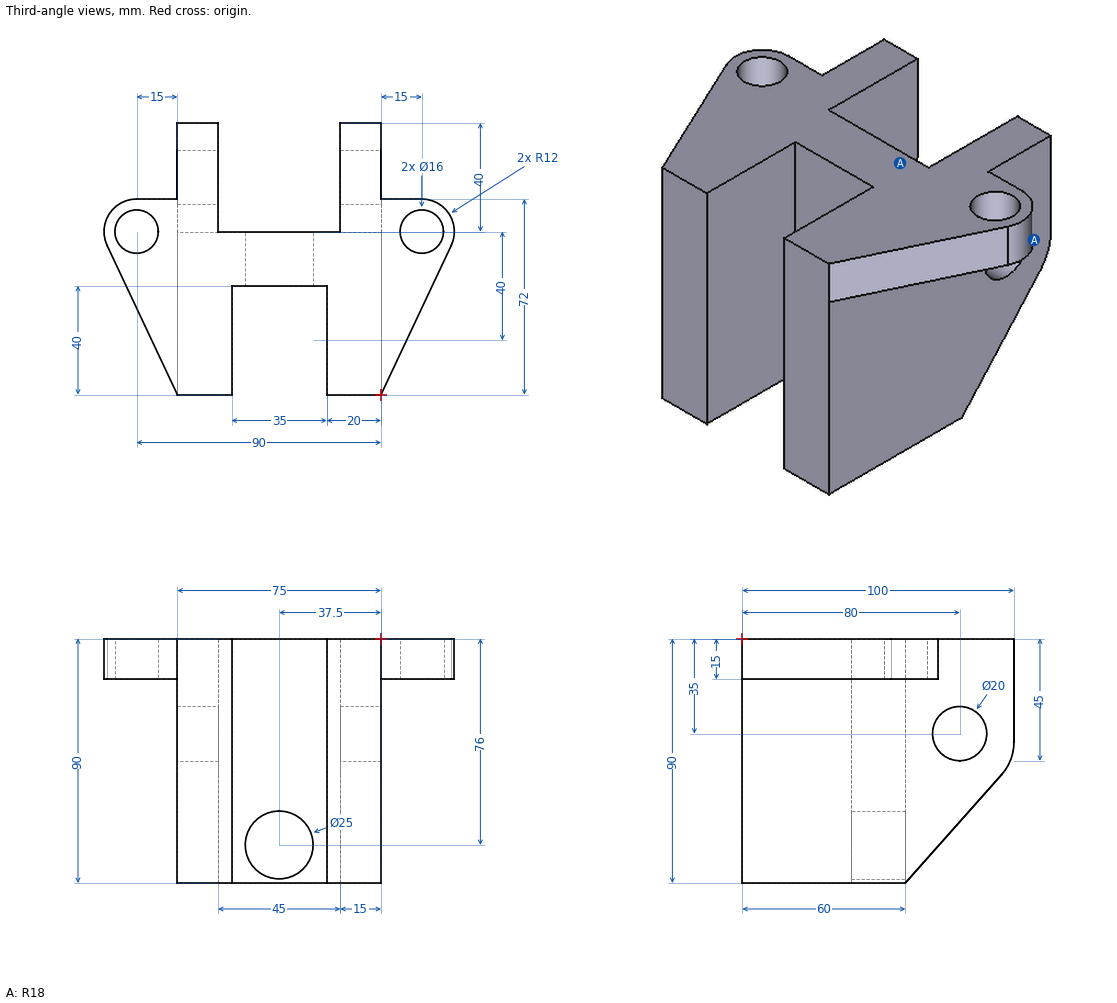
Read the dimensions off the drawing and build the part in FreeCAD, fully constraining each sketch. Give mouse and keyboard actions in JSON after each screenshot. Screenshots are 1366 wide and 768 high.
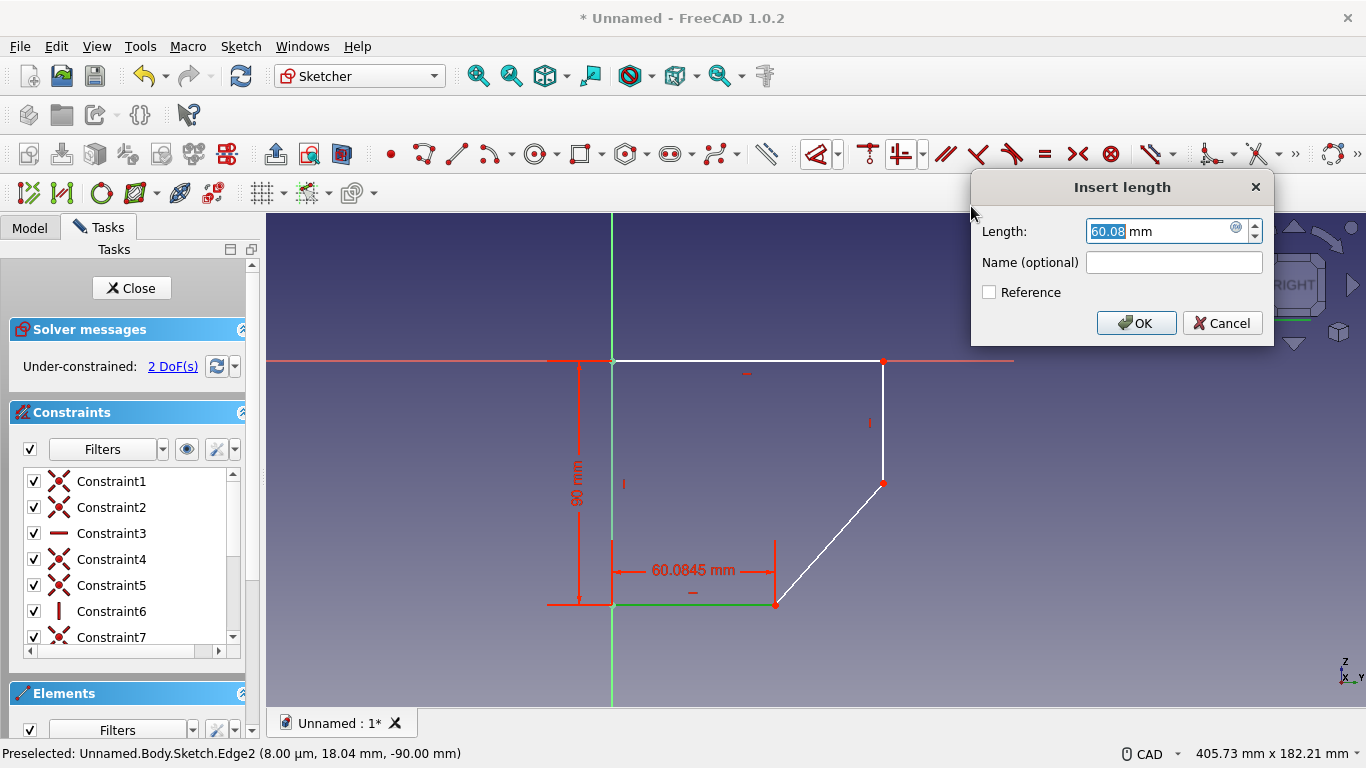
{"action": "type", "text": "60"}
{"action": "key", "text": "Return"}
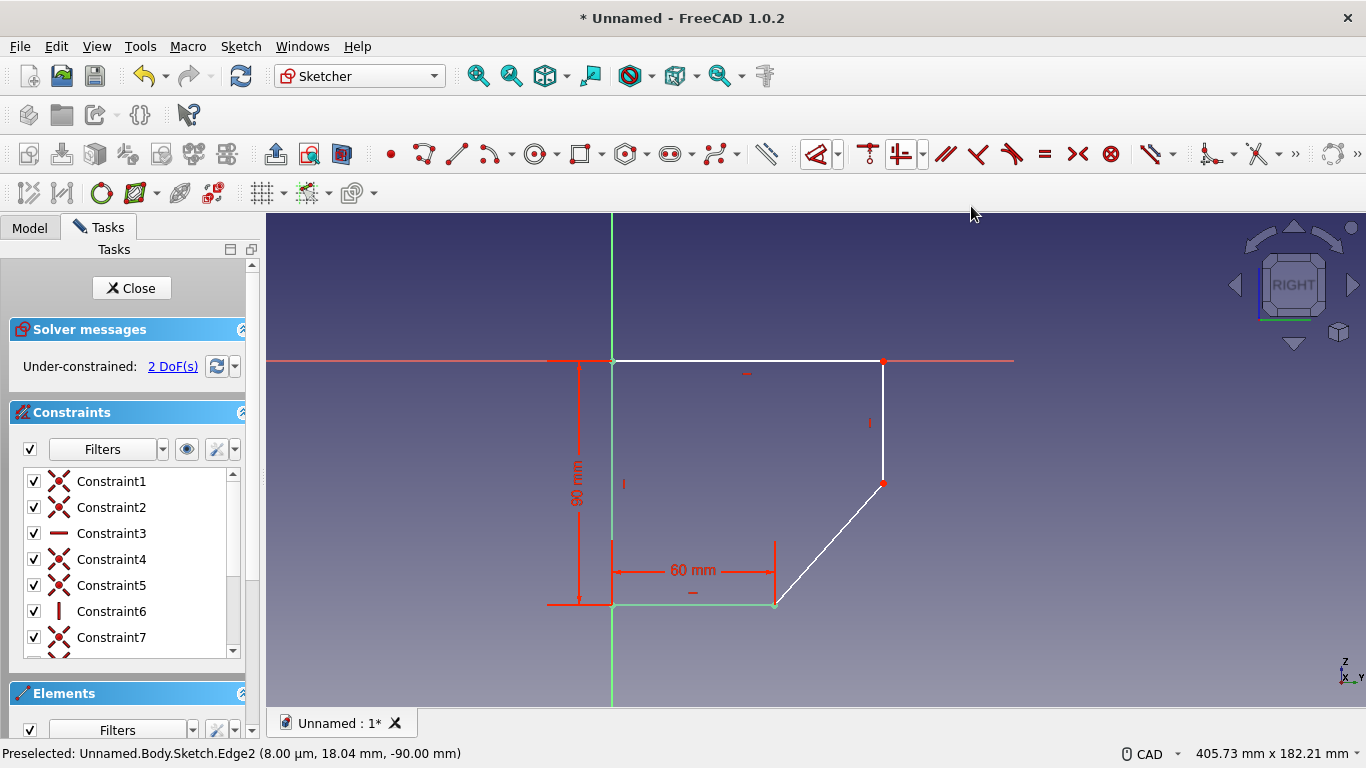
{"action": "left_click", "coordinate": [883, 447]}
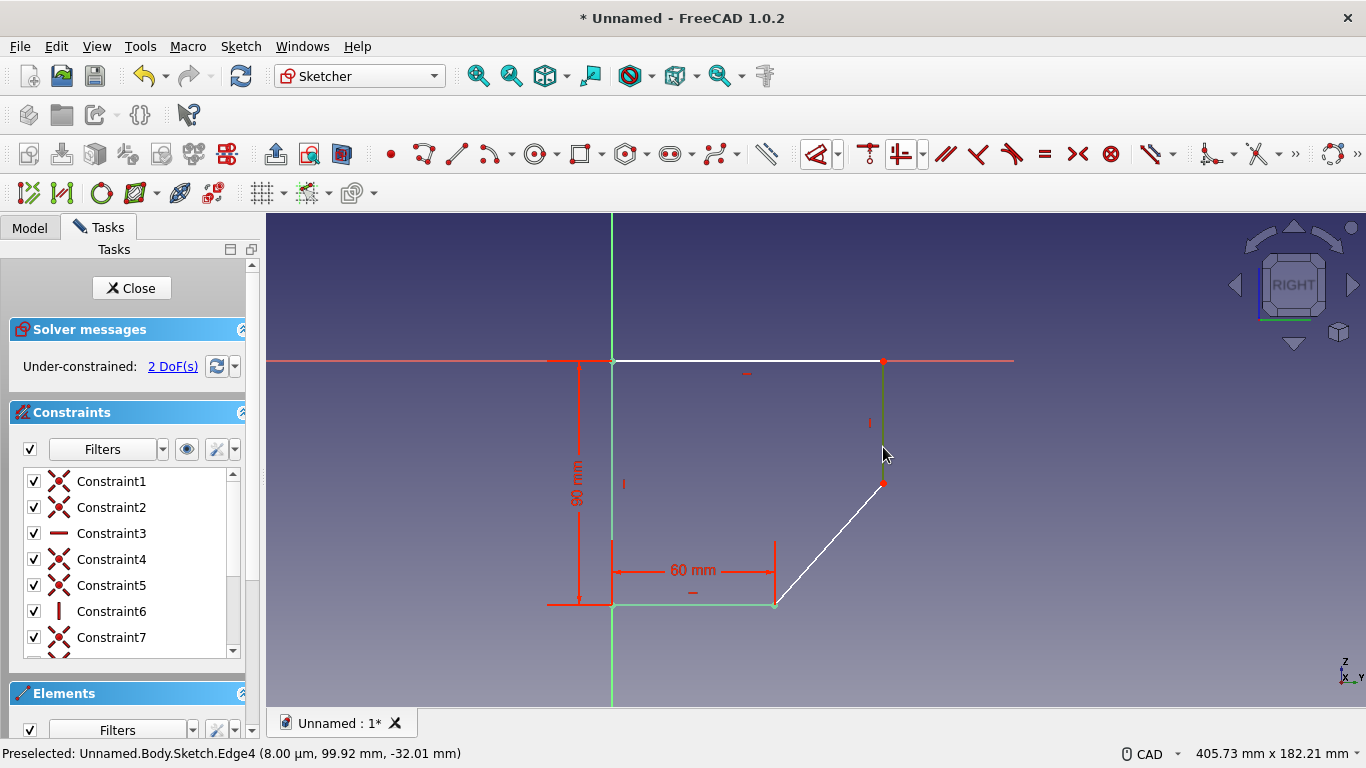
{"action": "key", "text": "i"}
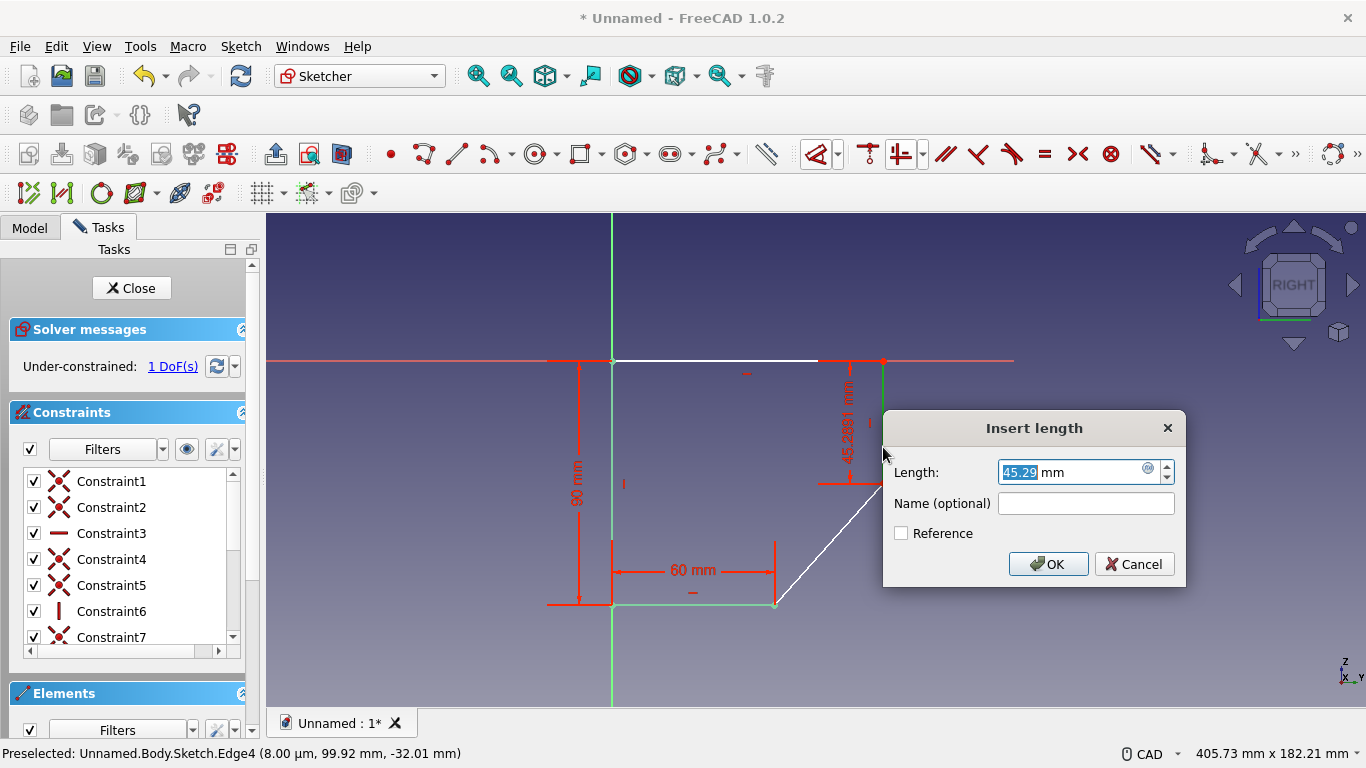
{"action": "type", "text": "45"}
{"action": "key", "text": "Return"}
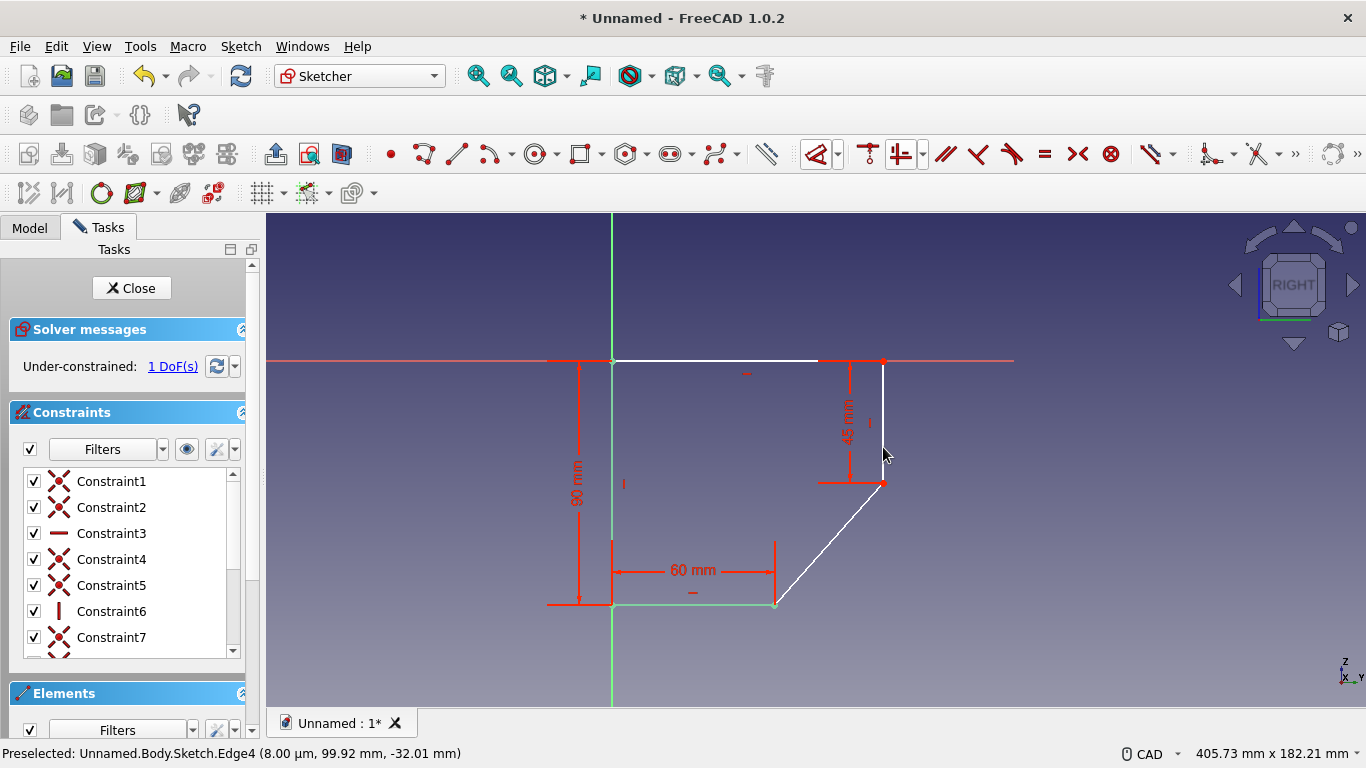
{"action": "left_click", "coordinate": [802, 361]}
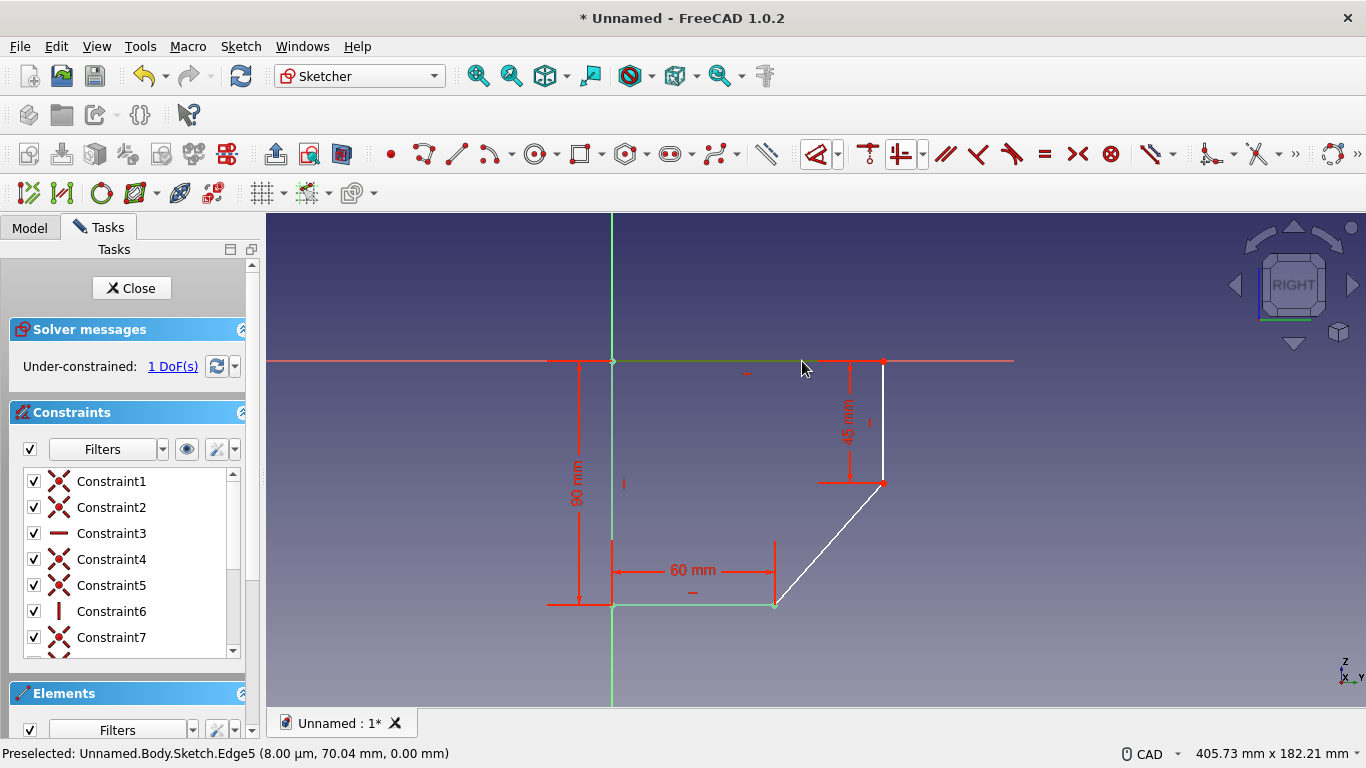
{"action": "key", "text": "l"}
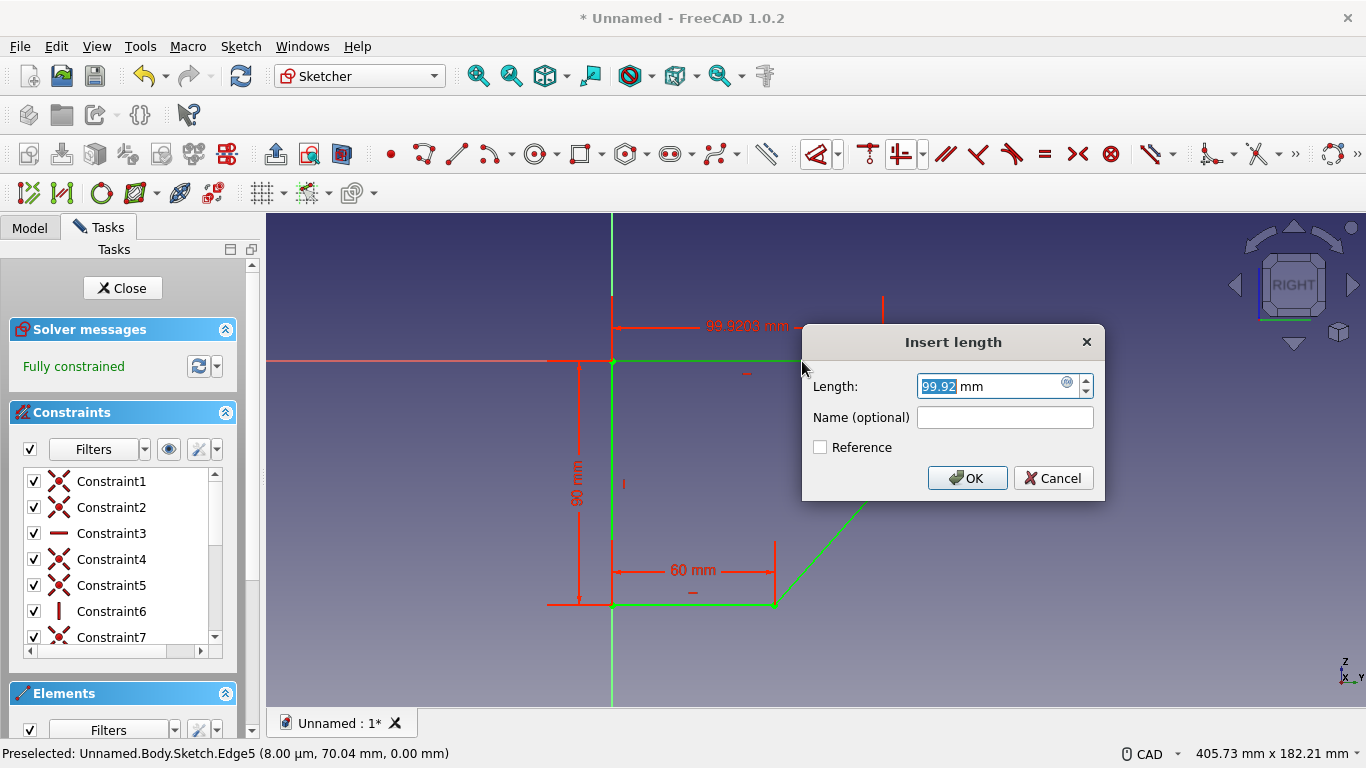
{"action": "type", "text": "100"}
{"action": "key", "text": "Return"}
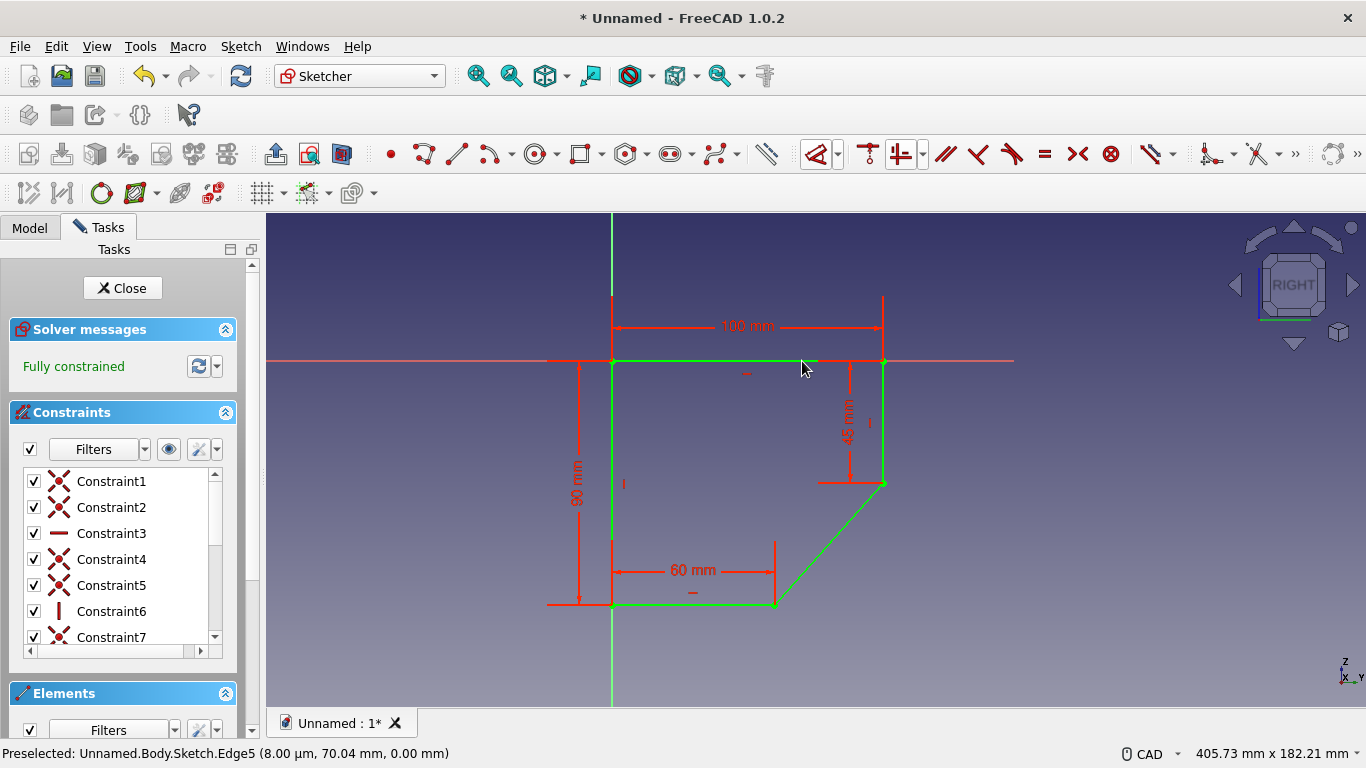
{"action": "left_click", "coordinate": [123, 288]}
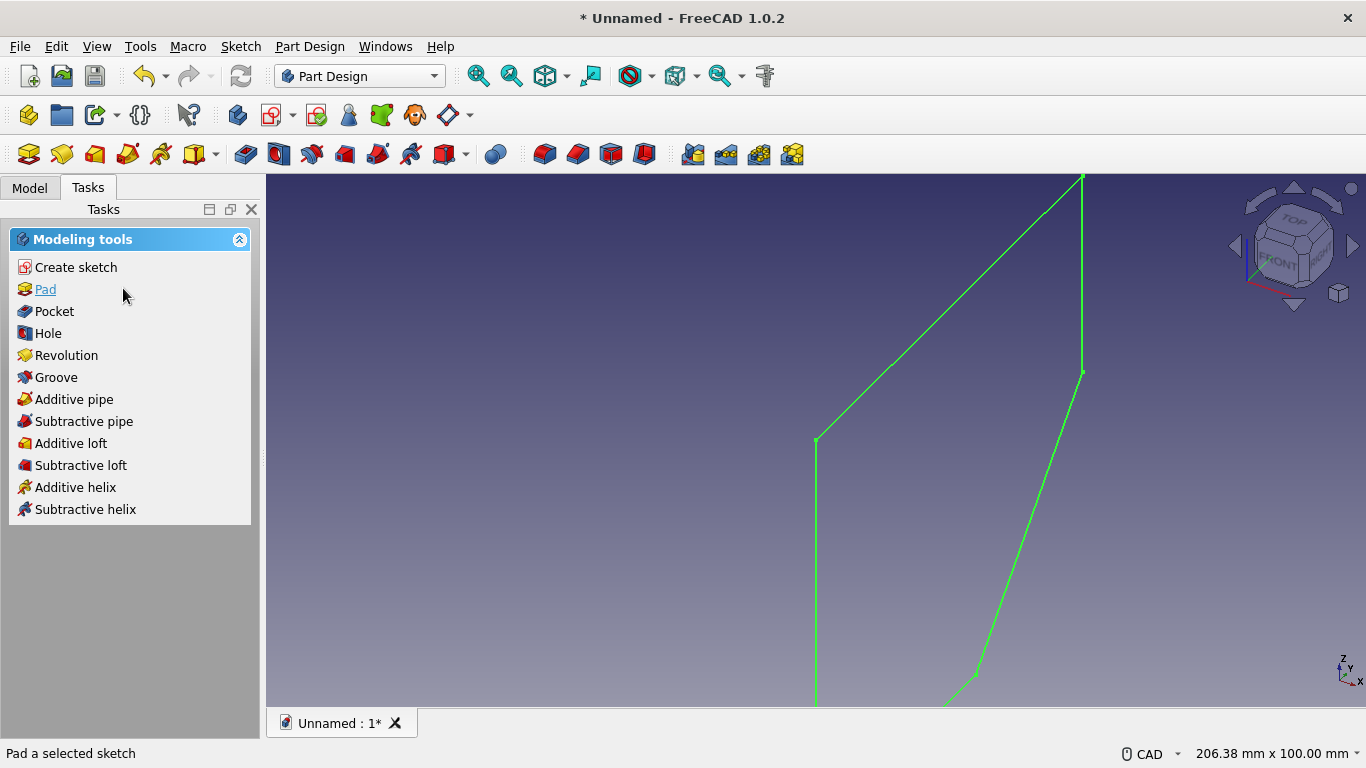
{"action": "left_click", "coordinate": [29, 154]}